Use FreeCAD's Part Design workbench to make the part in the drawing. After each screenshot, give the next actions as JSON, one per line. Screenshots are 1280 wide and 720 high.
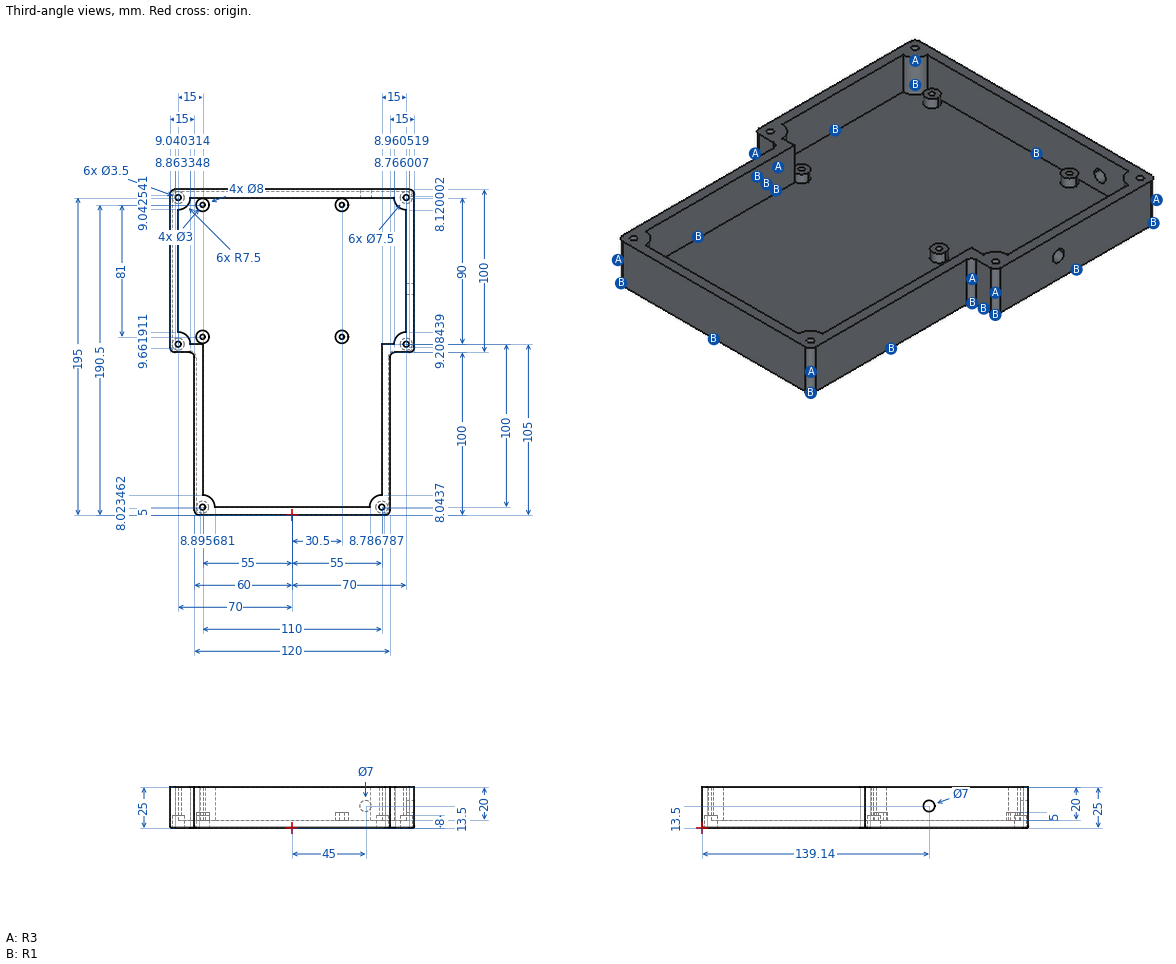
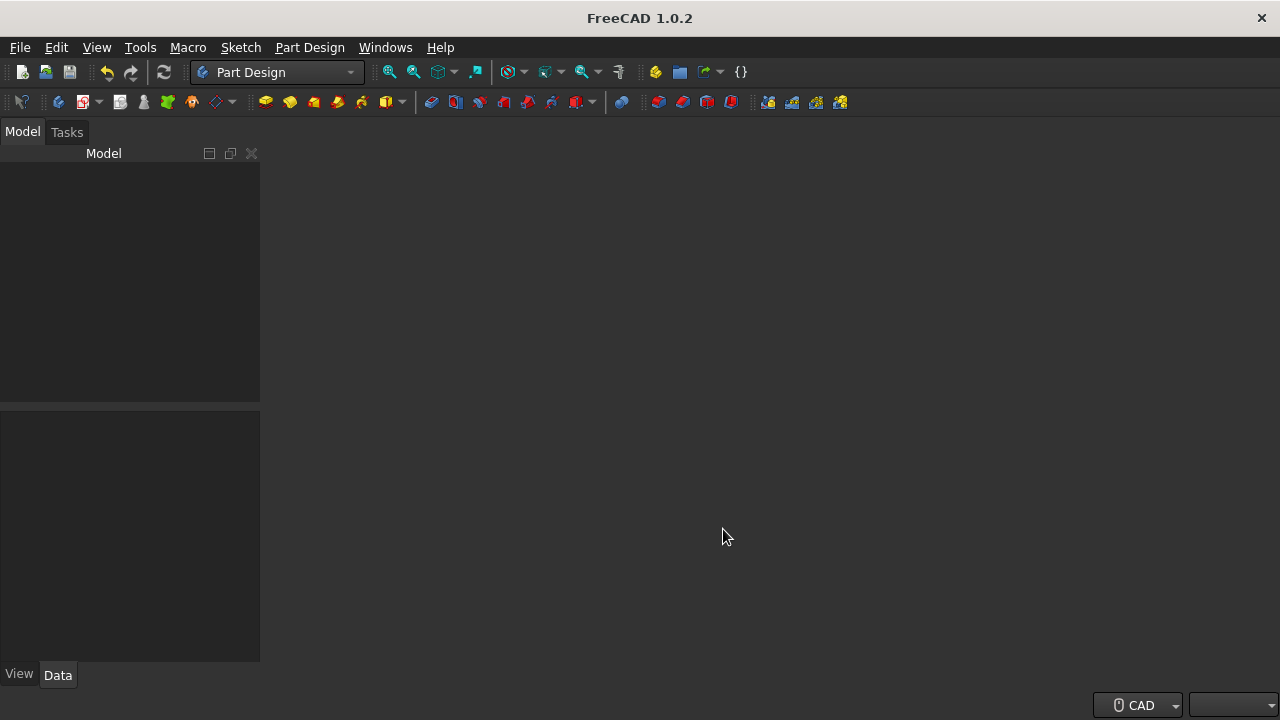
{"action": "key", "text": "ctrl+n"}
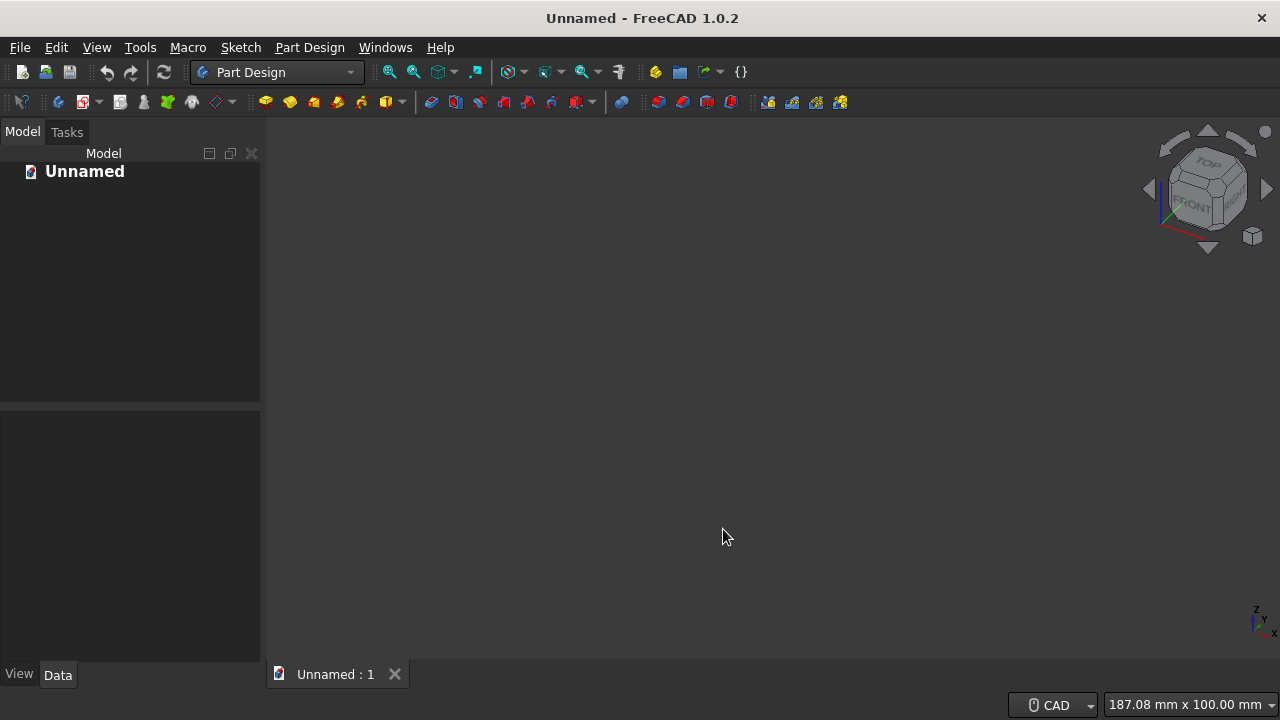
{"action": "left_click", "coordinate": [84, 102]}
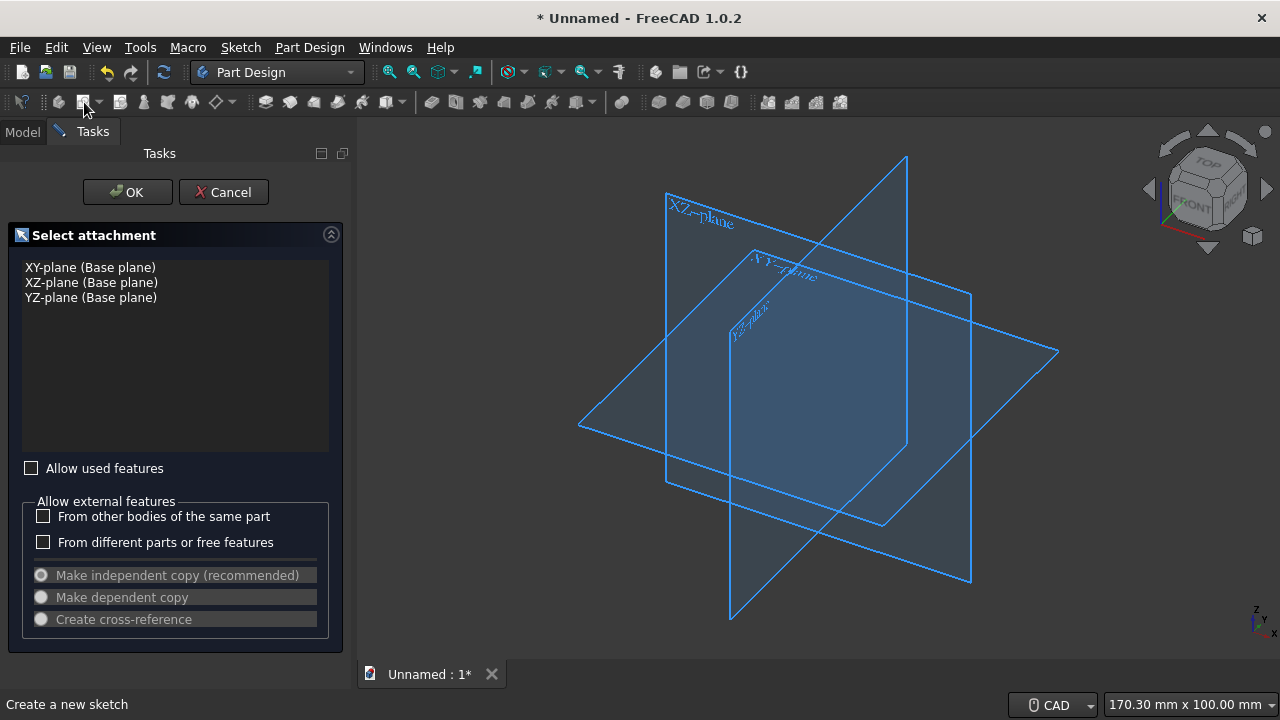
{"action": "left_click", "coordinate": [82, 268]}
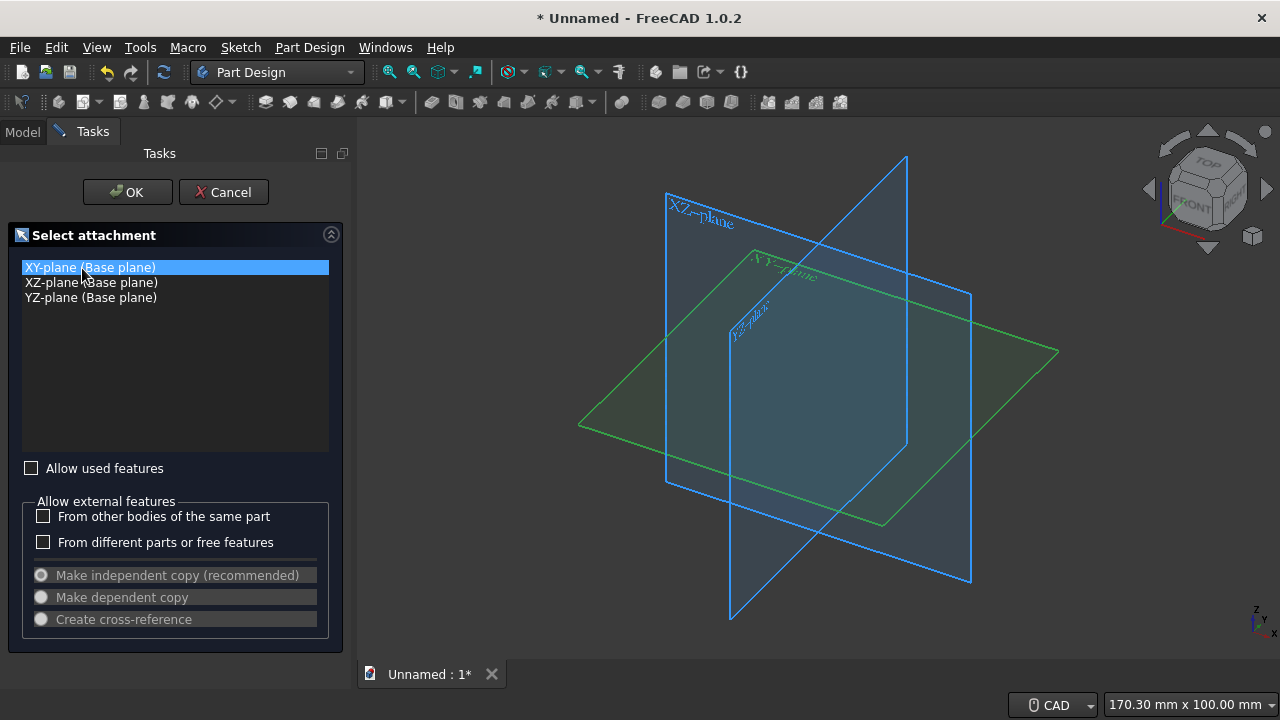
{"action": "left_click", "coordinate": [128, 192]}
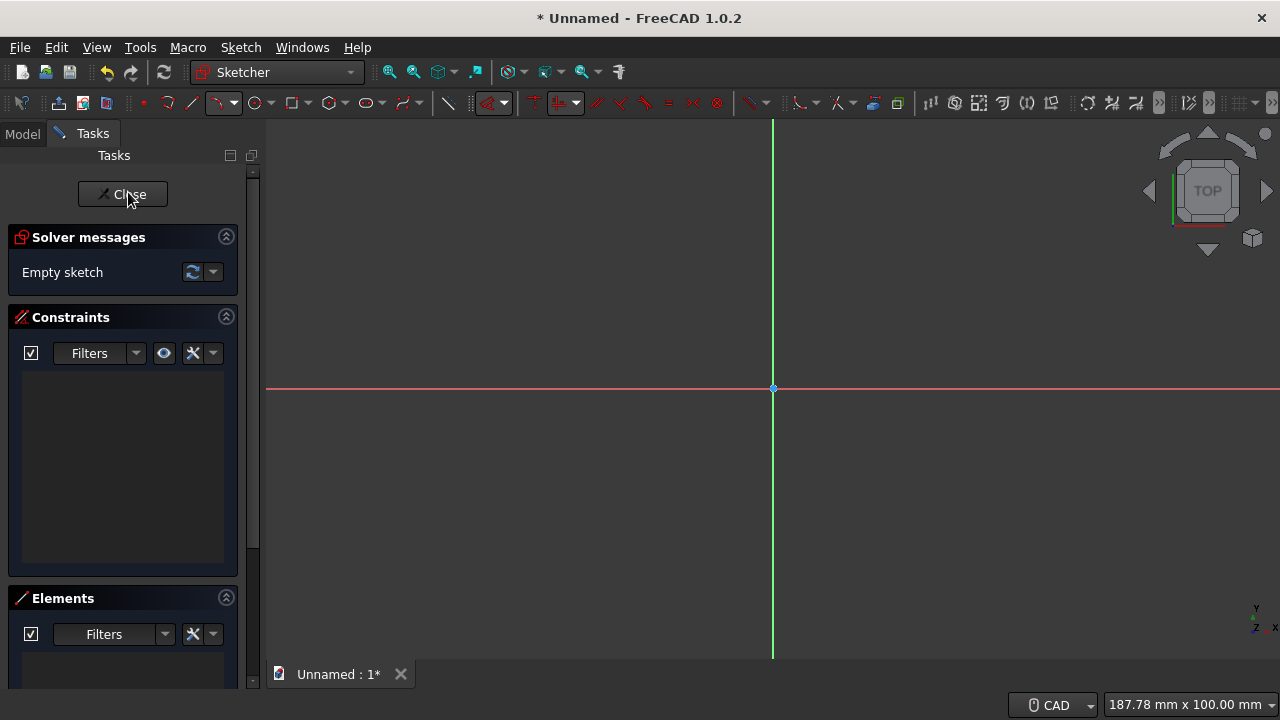
{"action": "scroll", "coordinate": [675, 622], "scroll_direction": "down", "scroll_amount": 6}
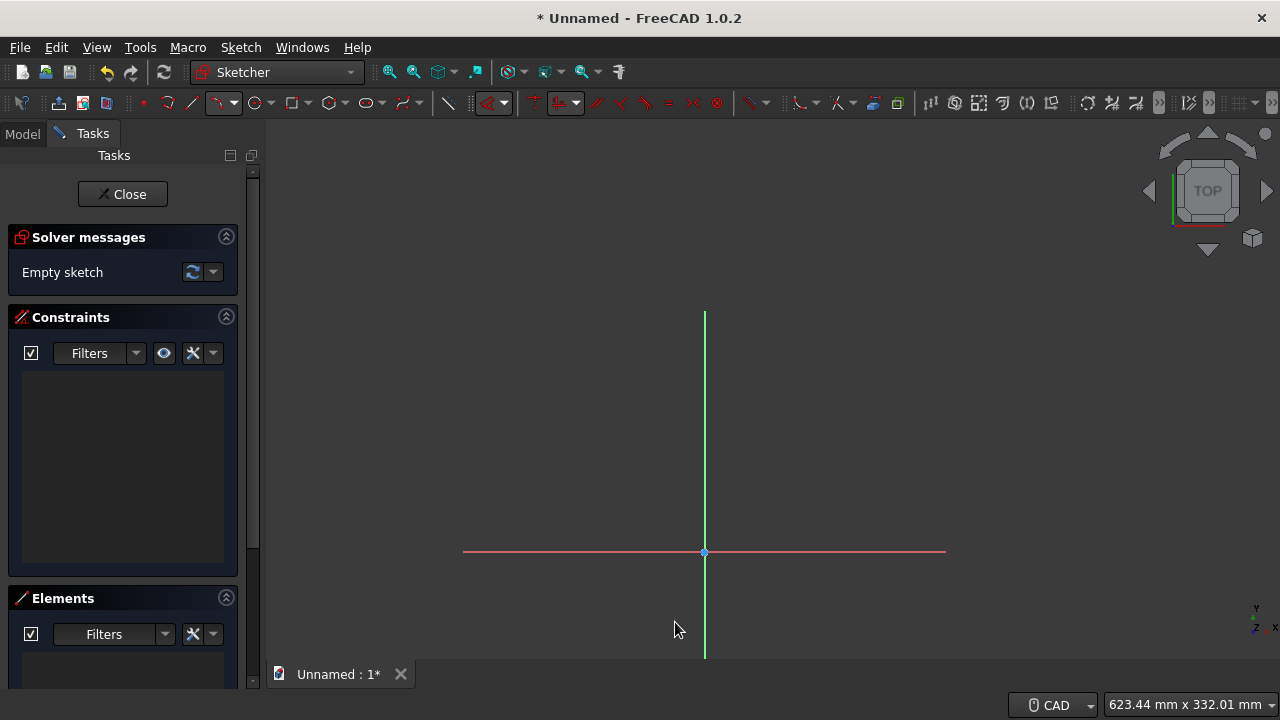
{"action": "key", "text": "g m"}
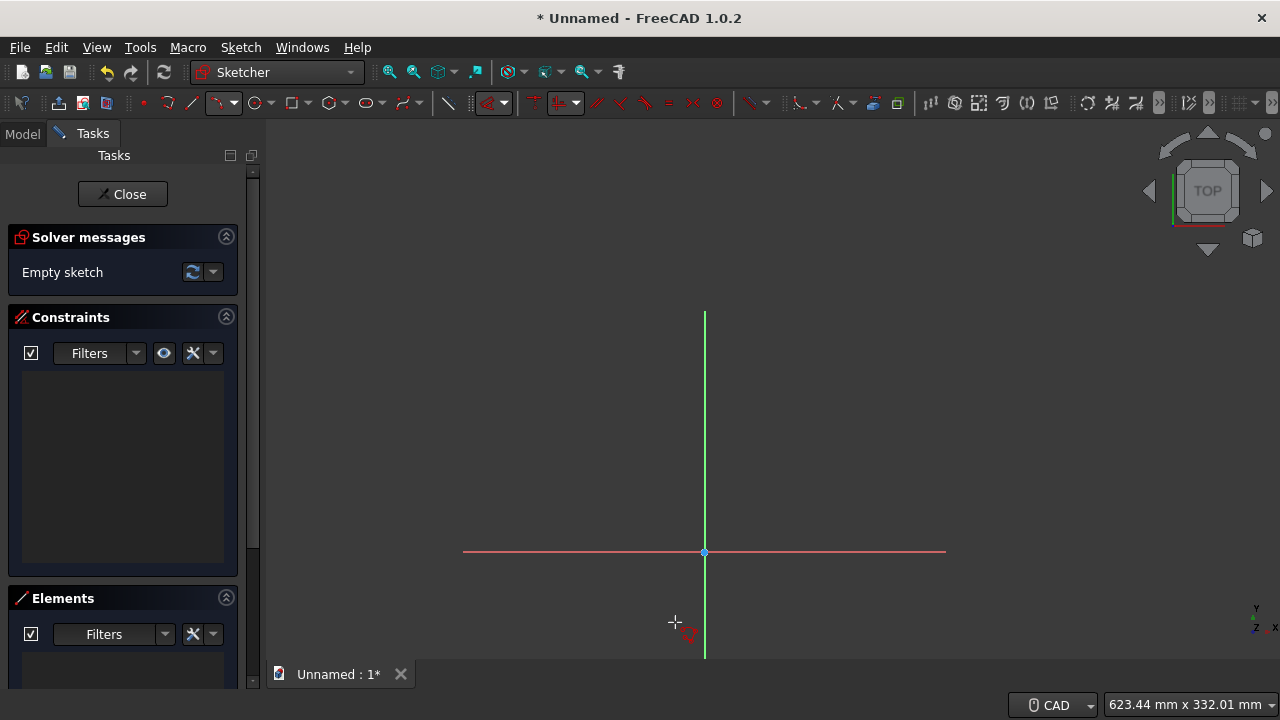
{"action": "left_click", "coordinate": [607, 552]}
{"action": "left_click", "coordinate": [802, 543]}
{"action": "left_click", "coordinate": [802, 390]}
{"action": "left_click", "coordinate": [827, 390]}
{"action": "left_click", "coordinate": [827, 227]}
{"action": "left_click", "coordinate": [583, 227]}
{"action": "left_click", "coordinate": [583, 390]}
{"action": "left_click", "coordinate": [607, 390]}
{"action": "left_click", "coordinate": [607, 552]}
{"action": "key", "text": "Escape"}
{"action": "key", "text": "Escape"}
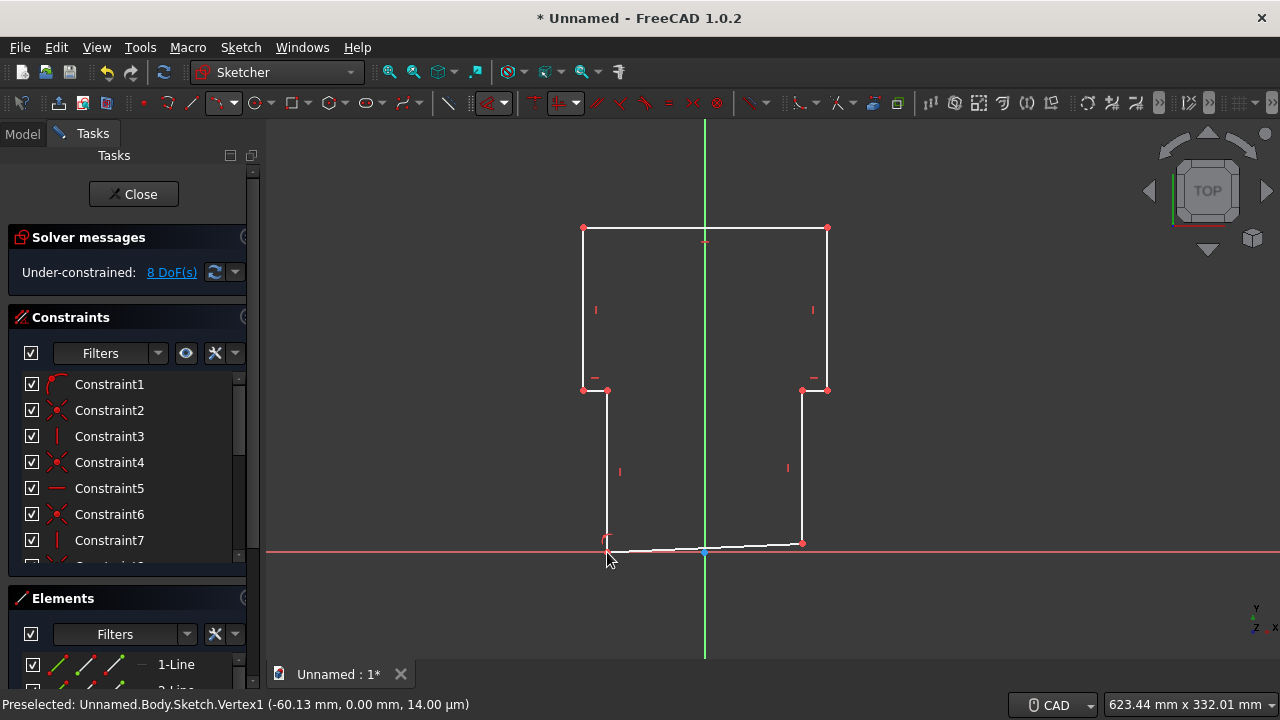
{"action": "left_click", "coordinate": [666, 550]}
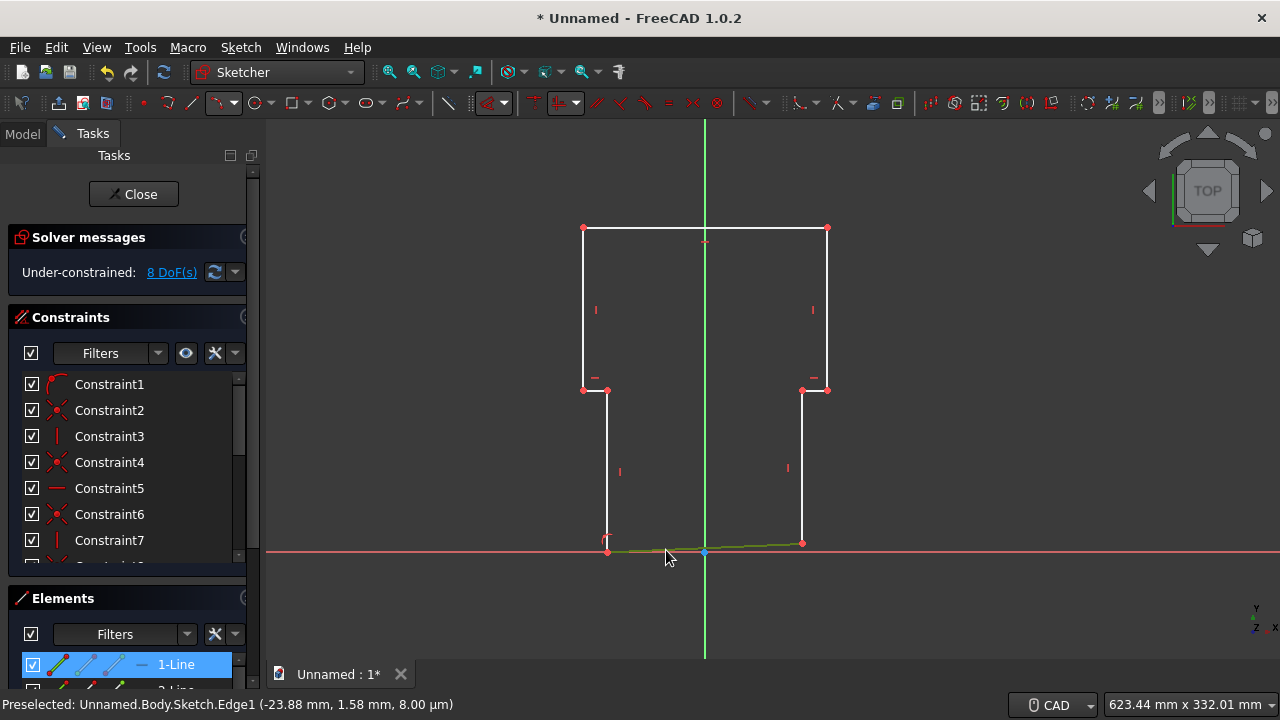
{"action": "key", "text": "h"}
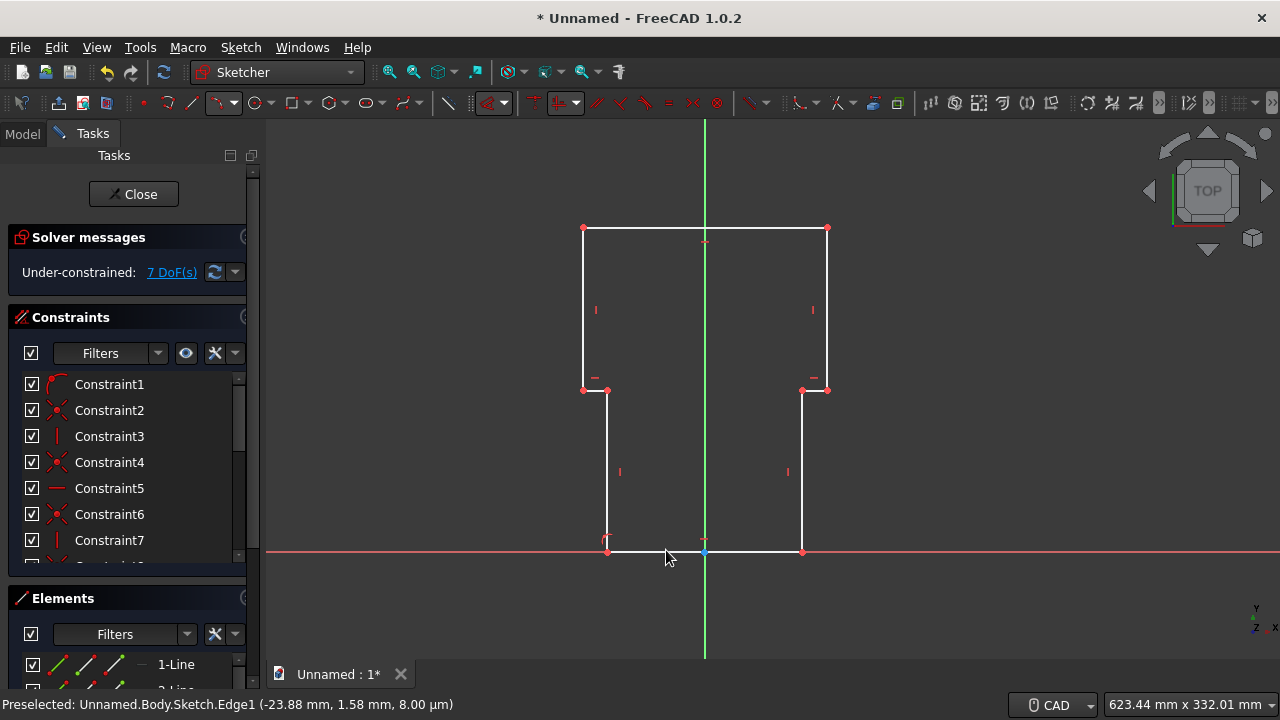
{"action": "left_click", "coordinate": [488, 104]}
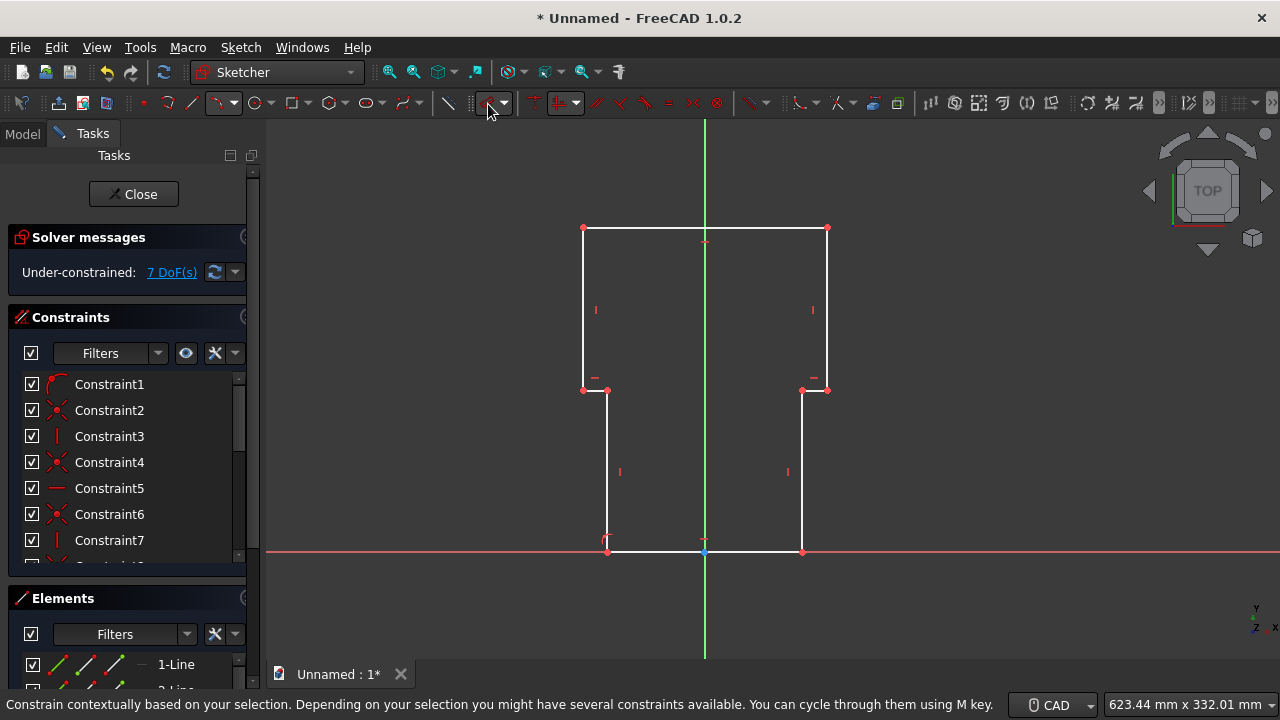
{"action": "scroll", "coordinate": [812, 391], "scroll_direction": "up", "scroll_amount": 3}